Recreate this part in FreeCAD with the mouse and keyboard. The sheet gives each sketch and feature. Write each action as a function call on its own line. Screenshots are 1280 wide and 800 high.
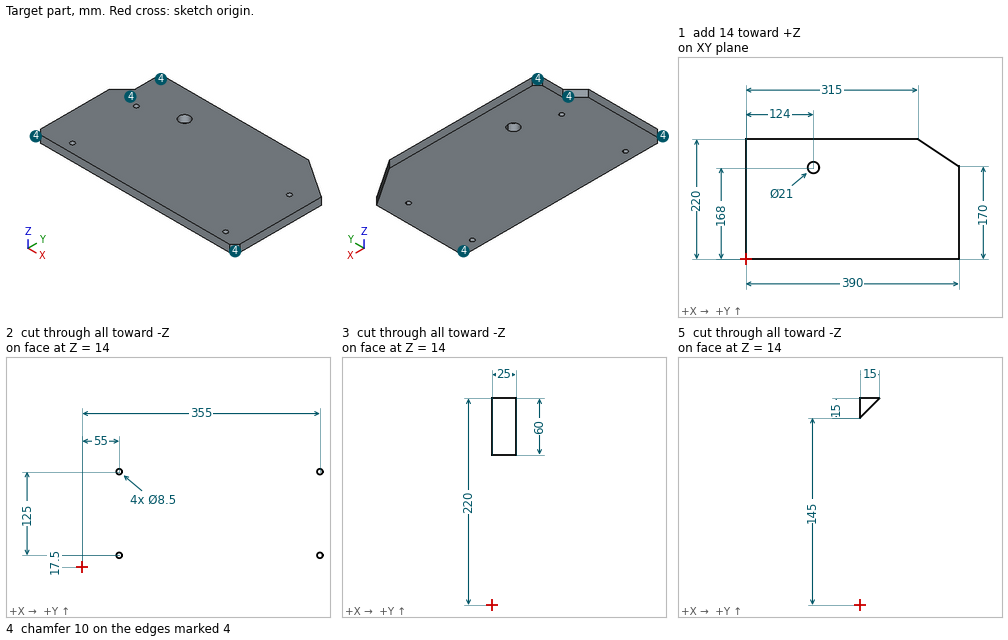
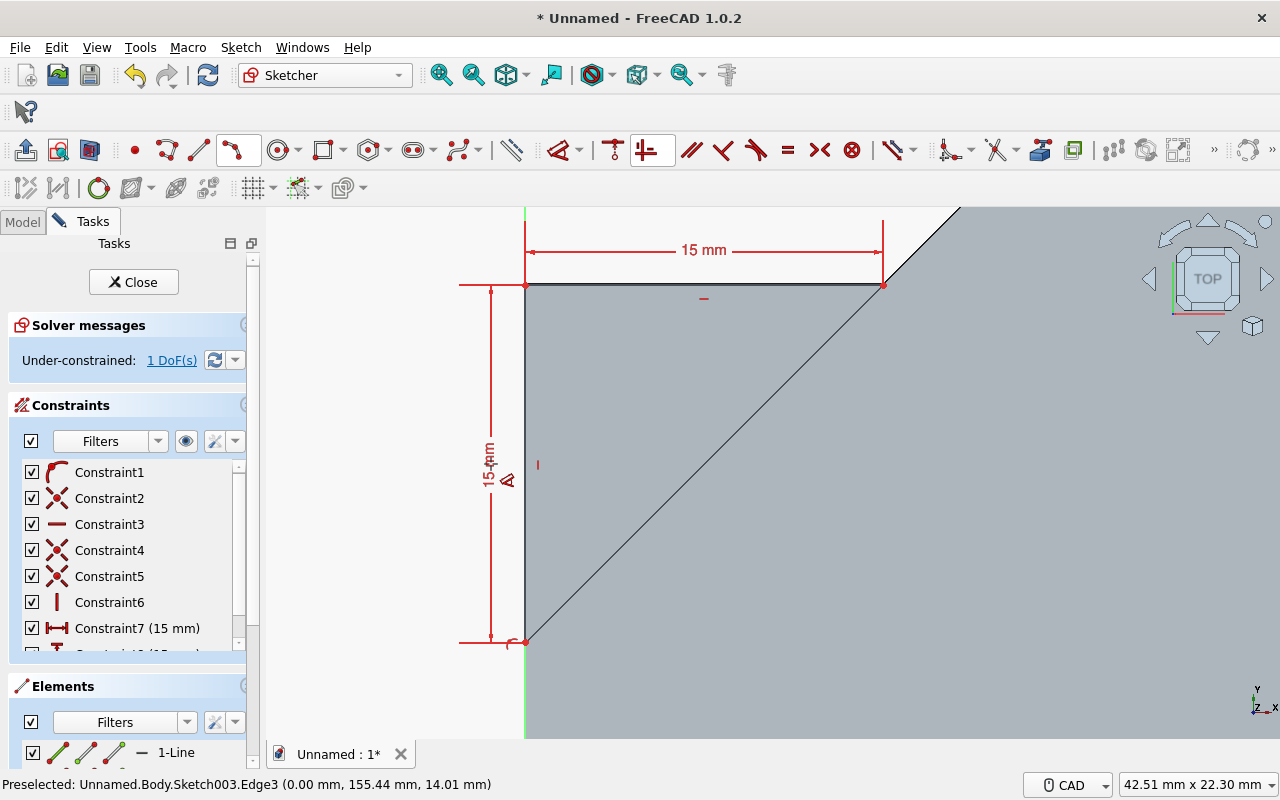
click(525, 643)
click(491, 677)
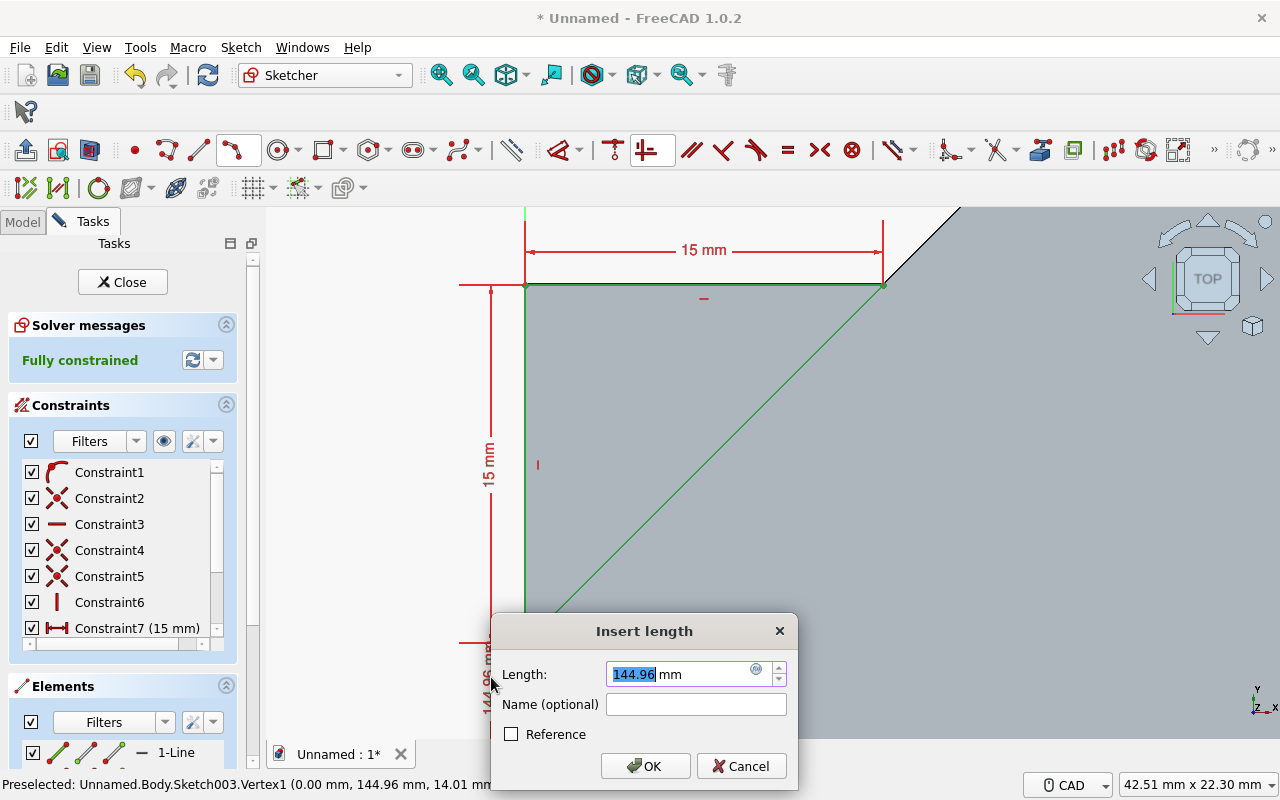
text(145)
key(Return)
key(Escape)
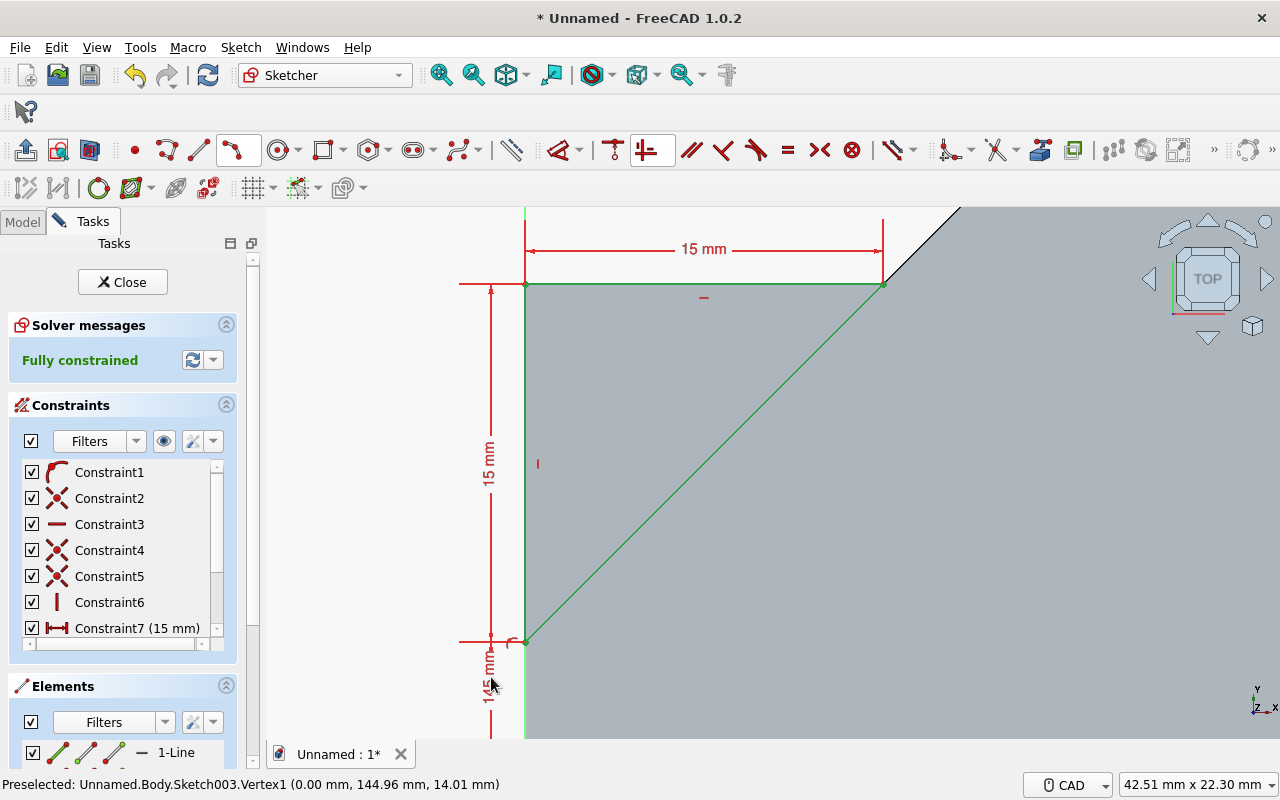
click(123, 282)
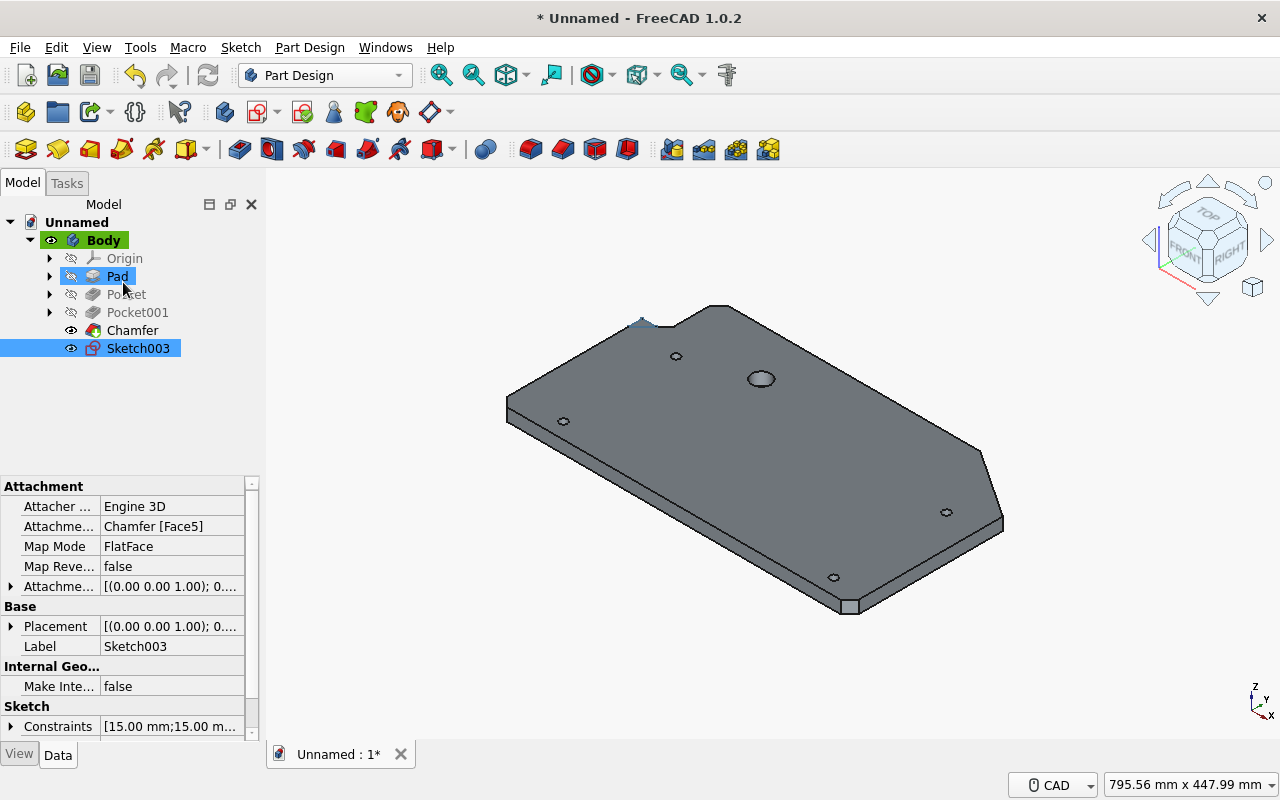
click(240, 150)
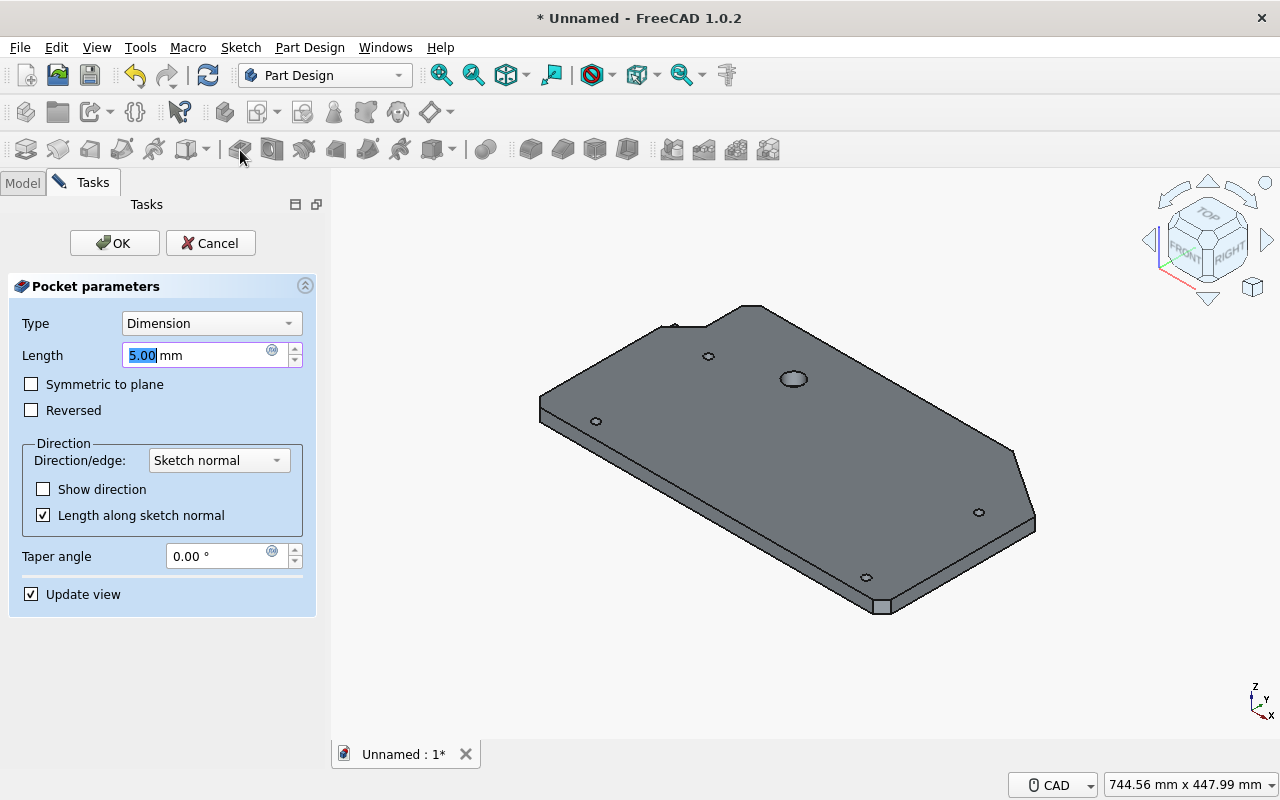
click(212, 324)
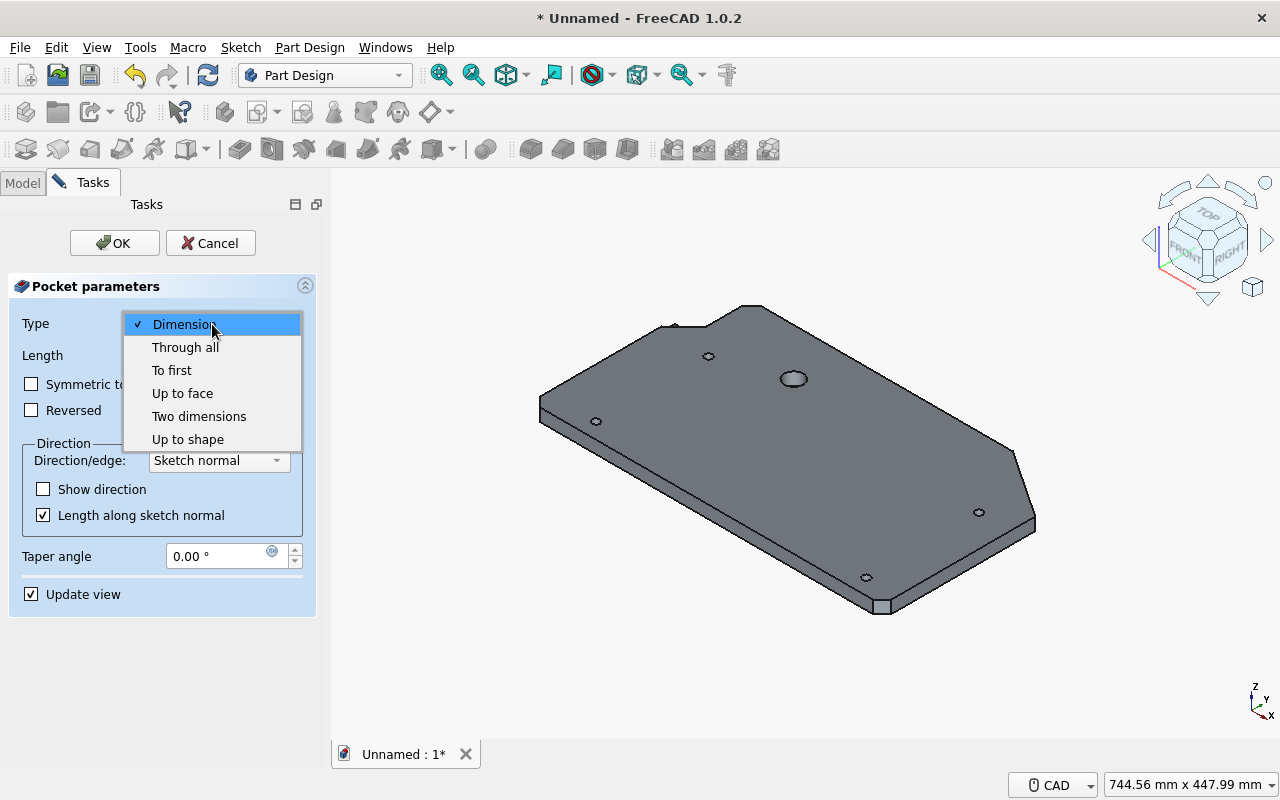
click(212, 348)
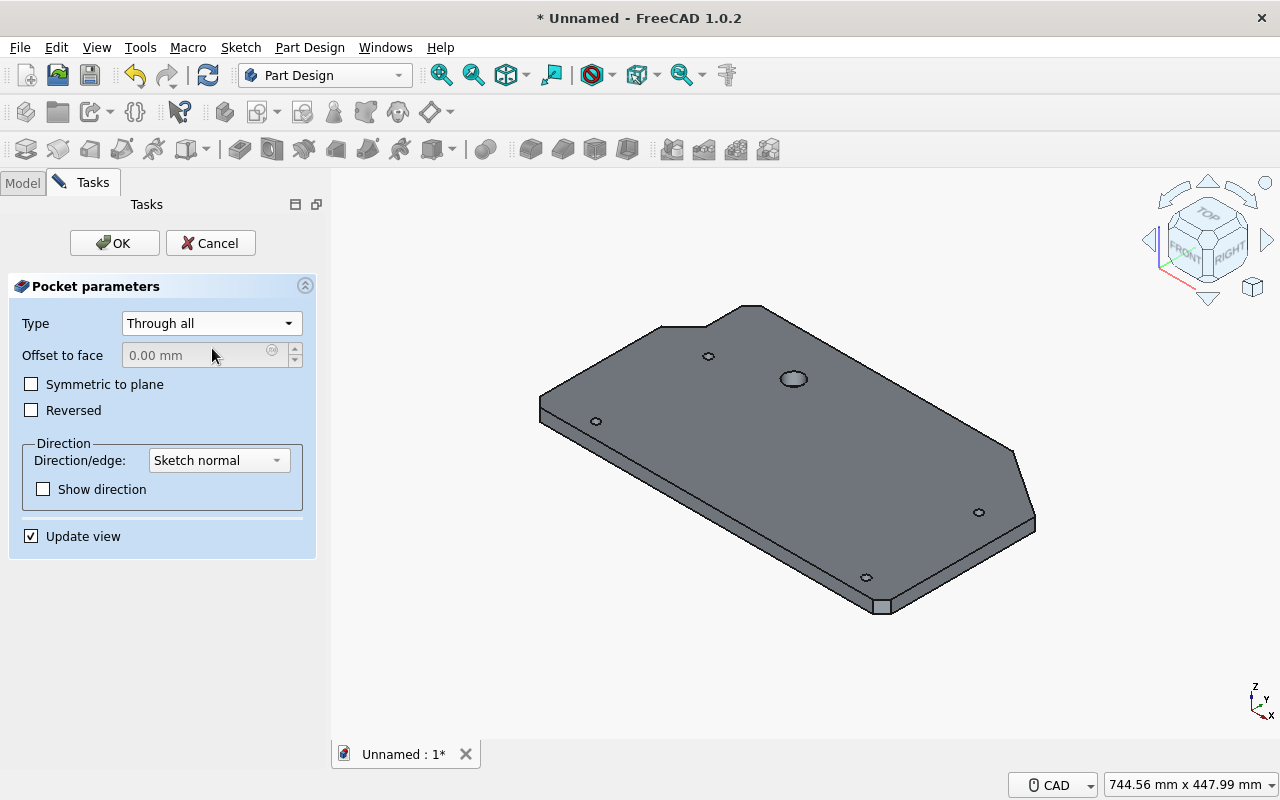
click(115, 243)